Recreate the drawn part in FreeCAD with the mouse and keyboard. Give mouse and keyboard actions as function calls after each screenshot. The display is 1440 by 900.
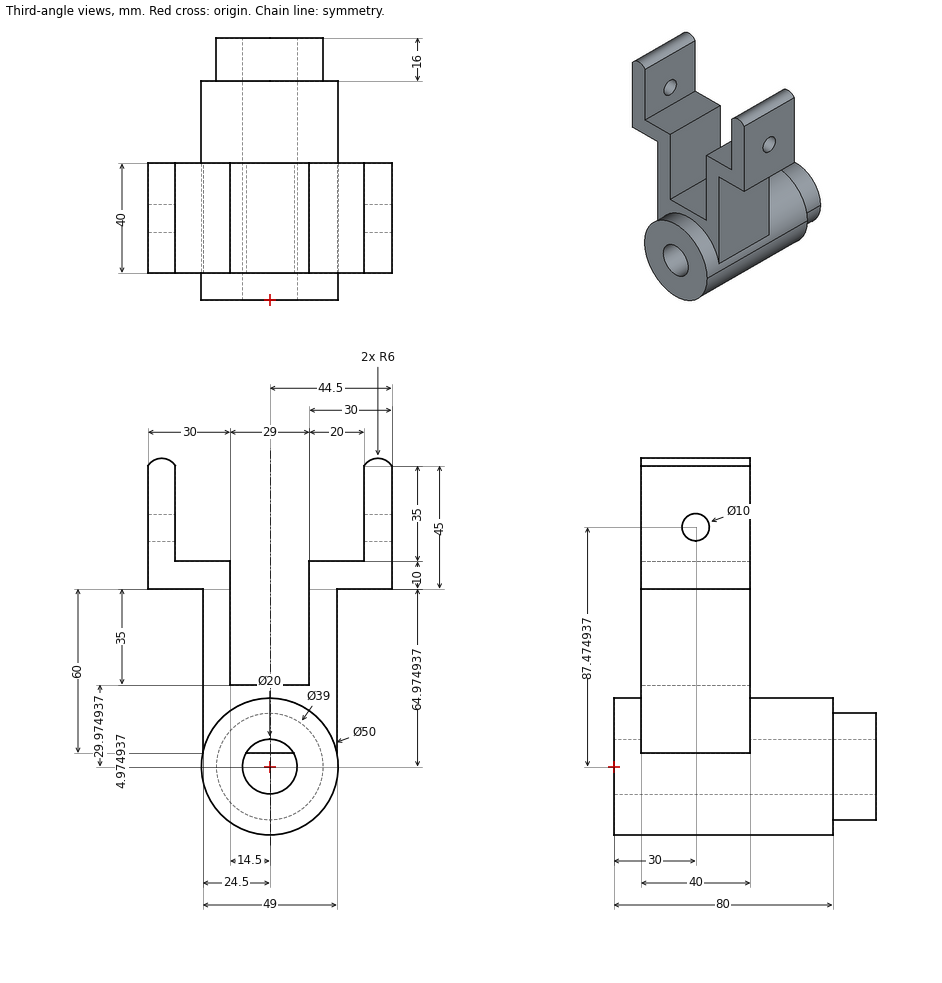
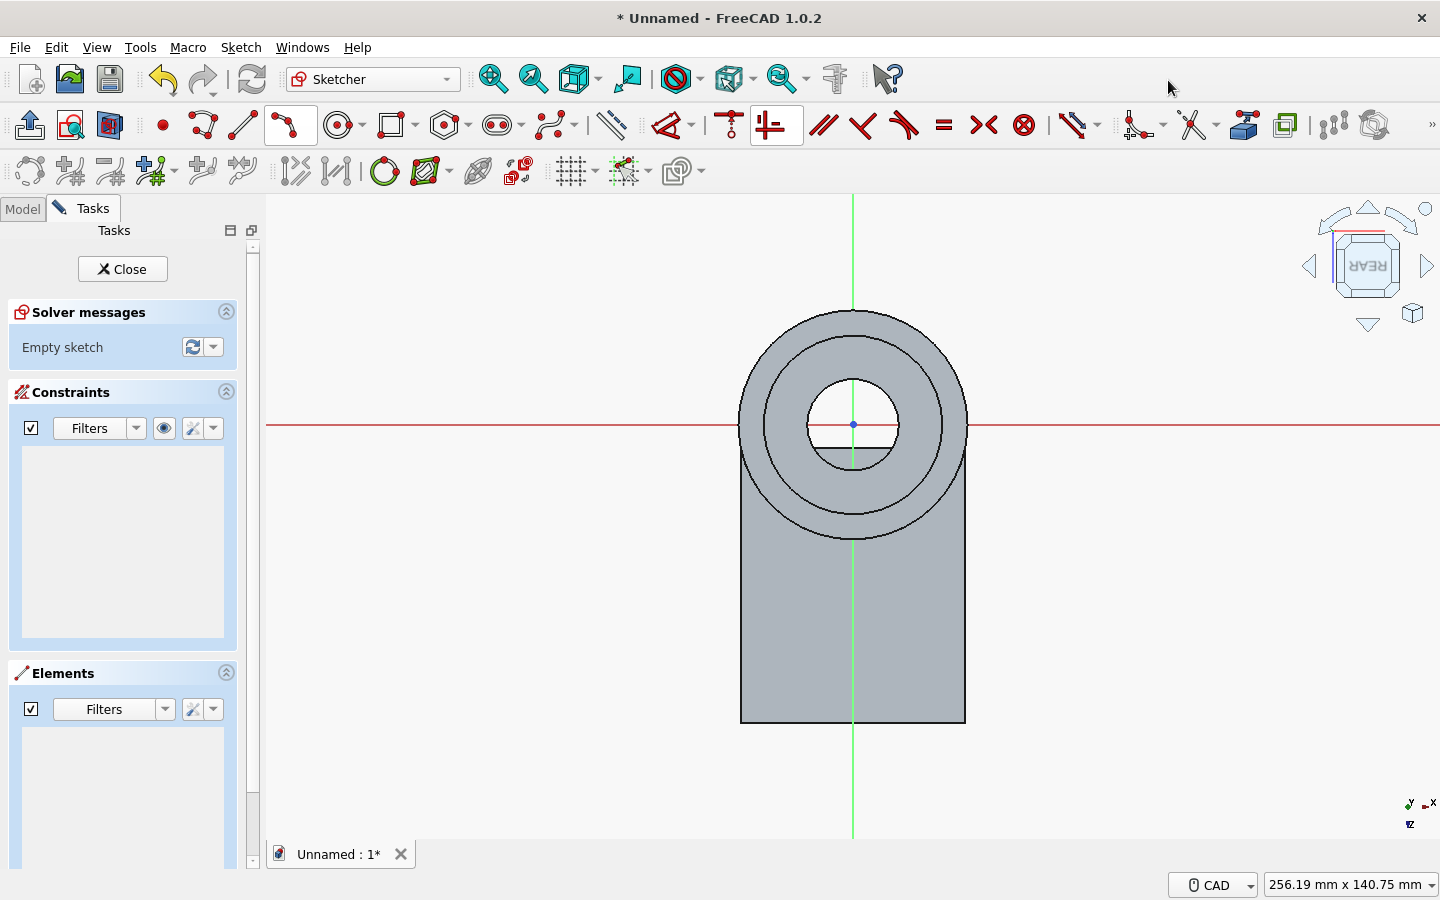
click(110, 126)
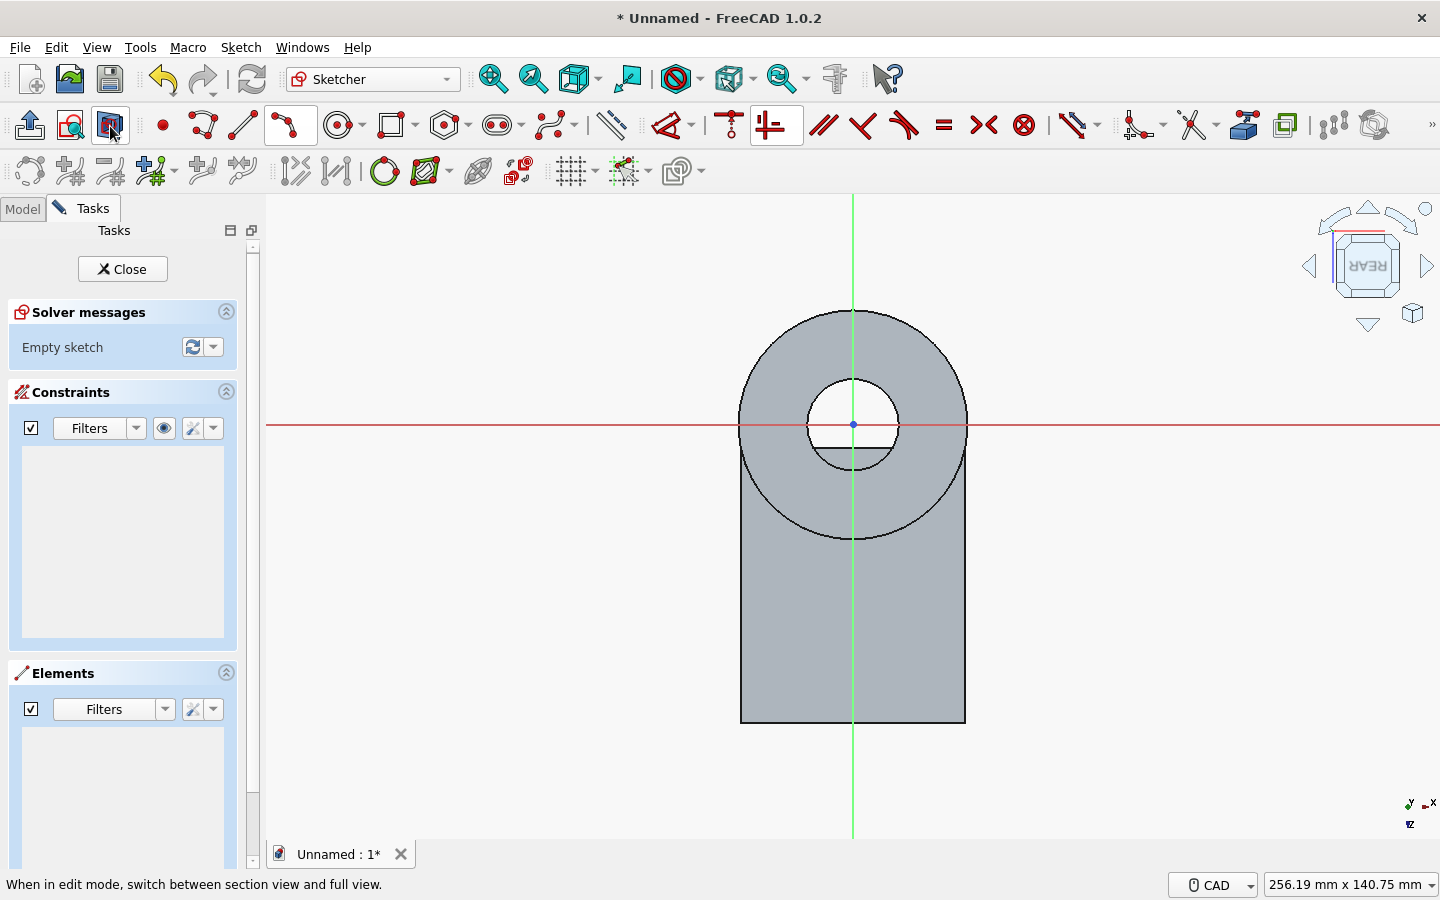
scroll(992, 690, up, 2)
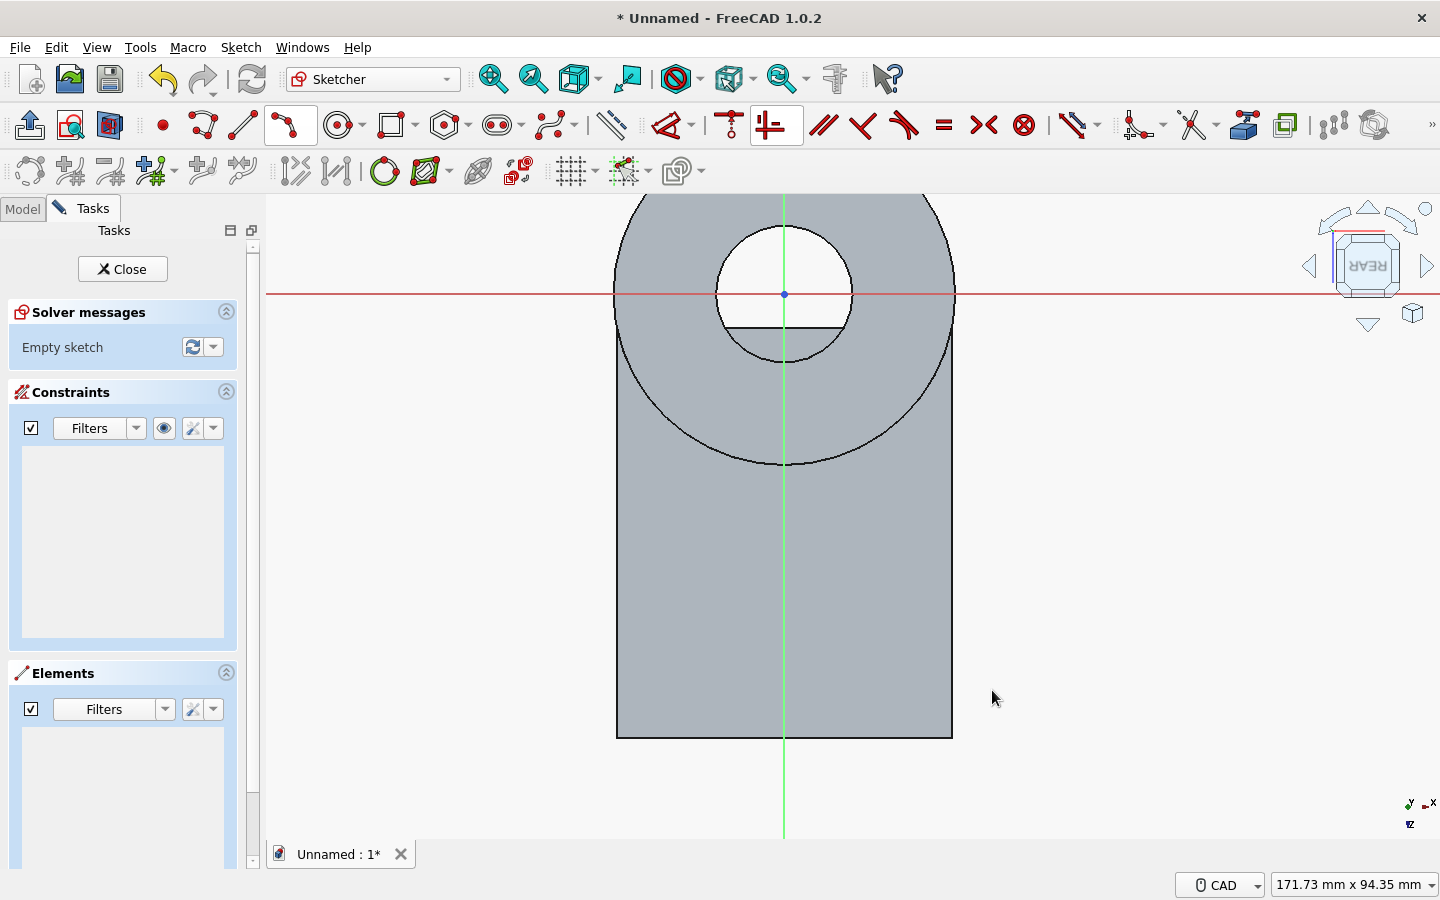
click(392, 126)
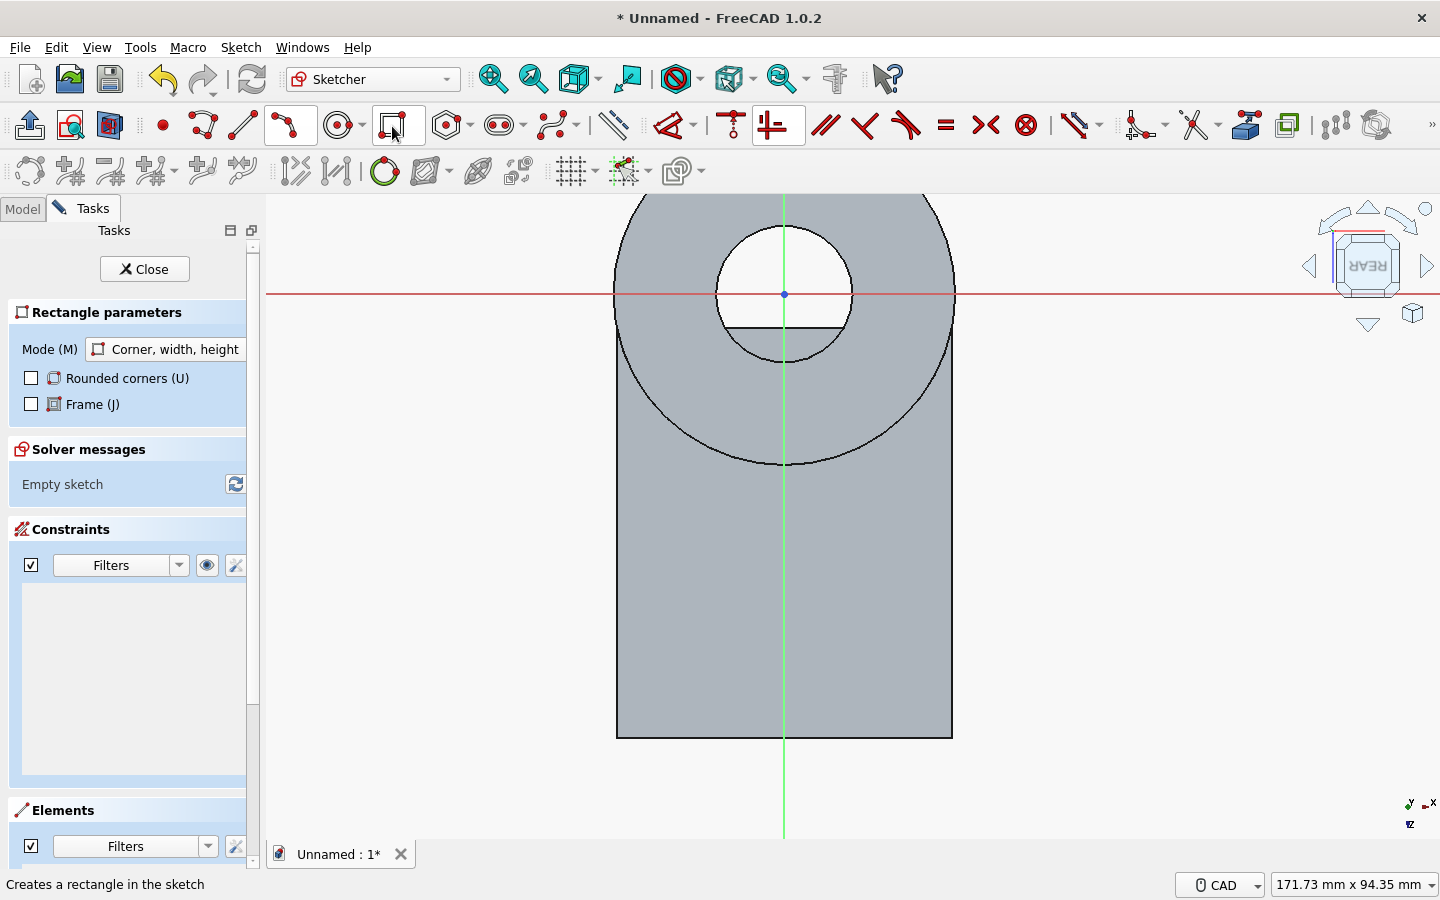
click(685, 499)
click(883, 738)
key(Escape)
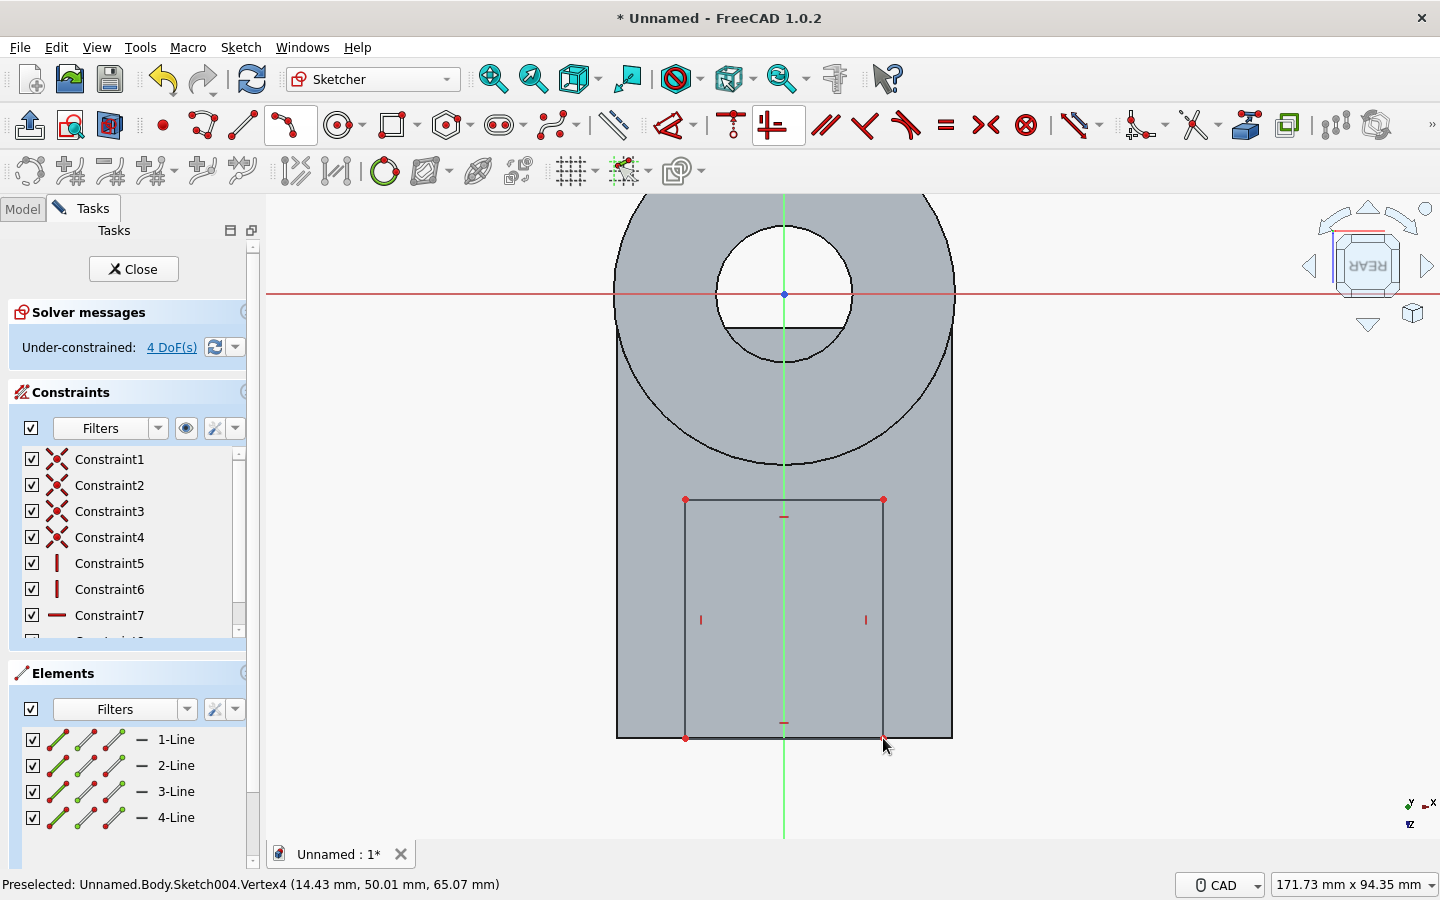
click(668, 126)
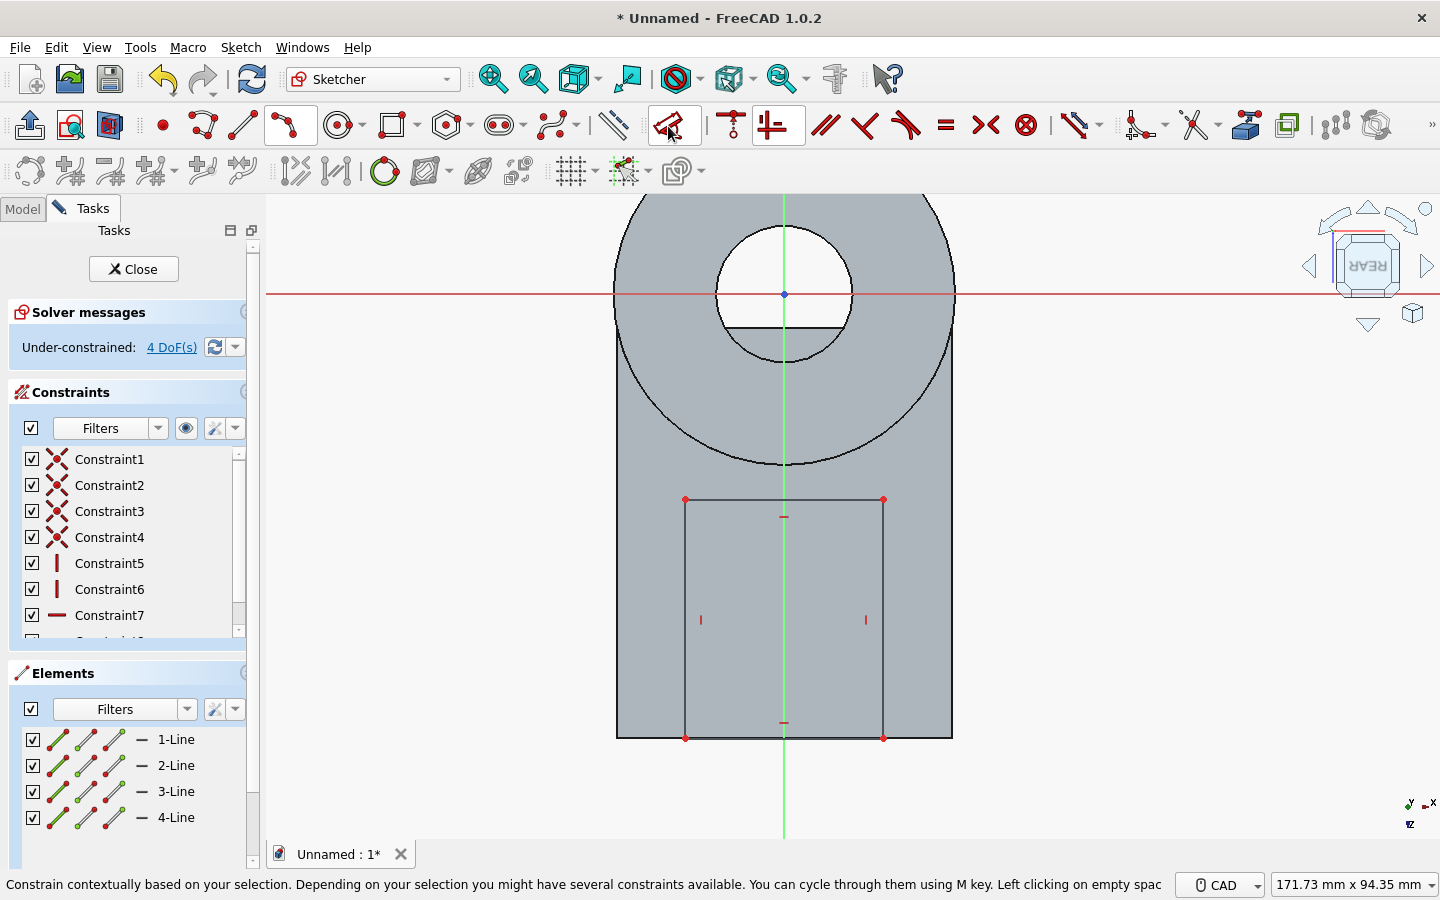
click(685, 572)
click(651, 619)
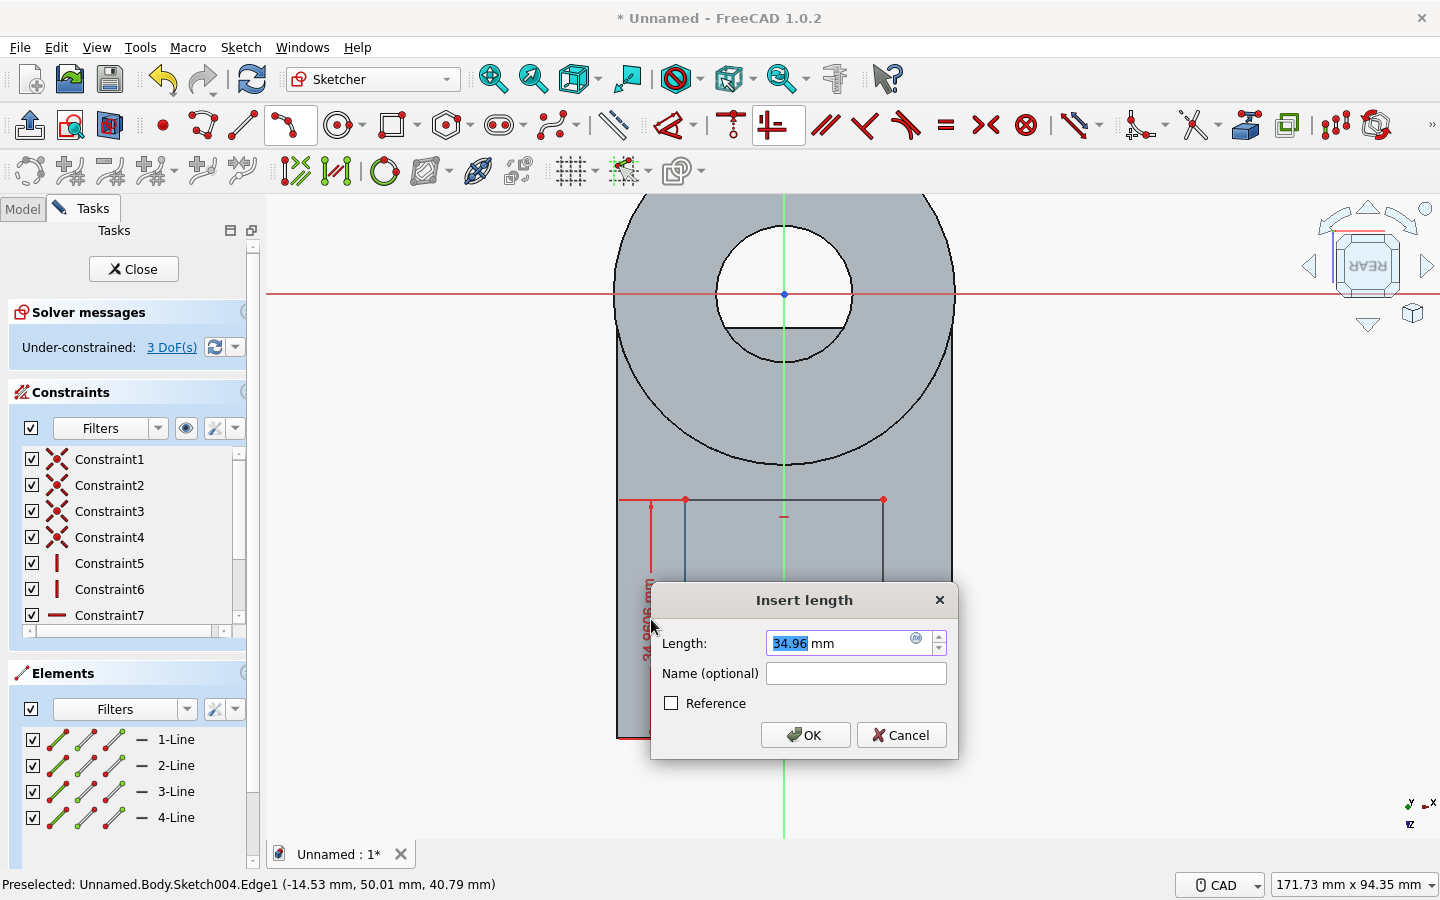
text(35)
key(Return)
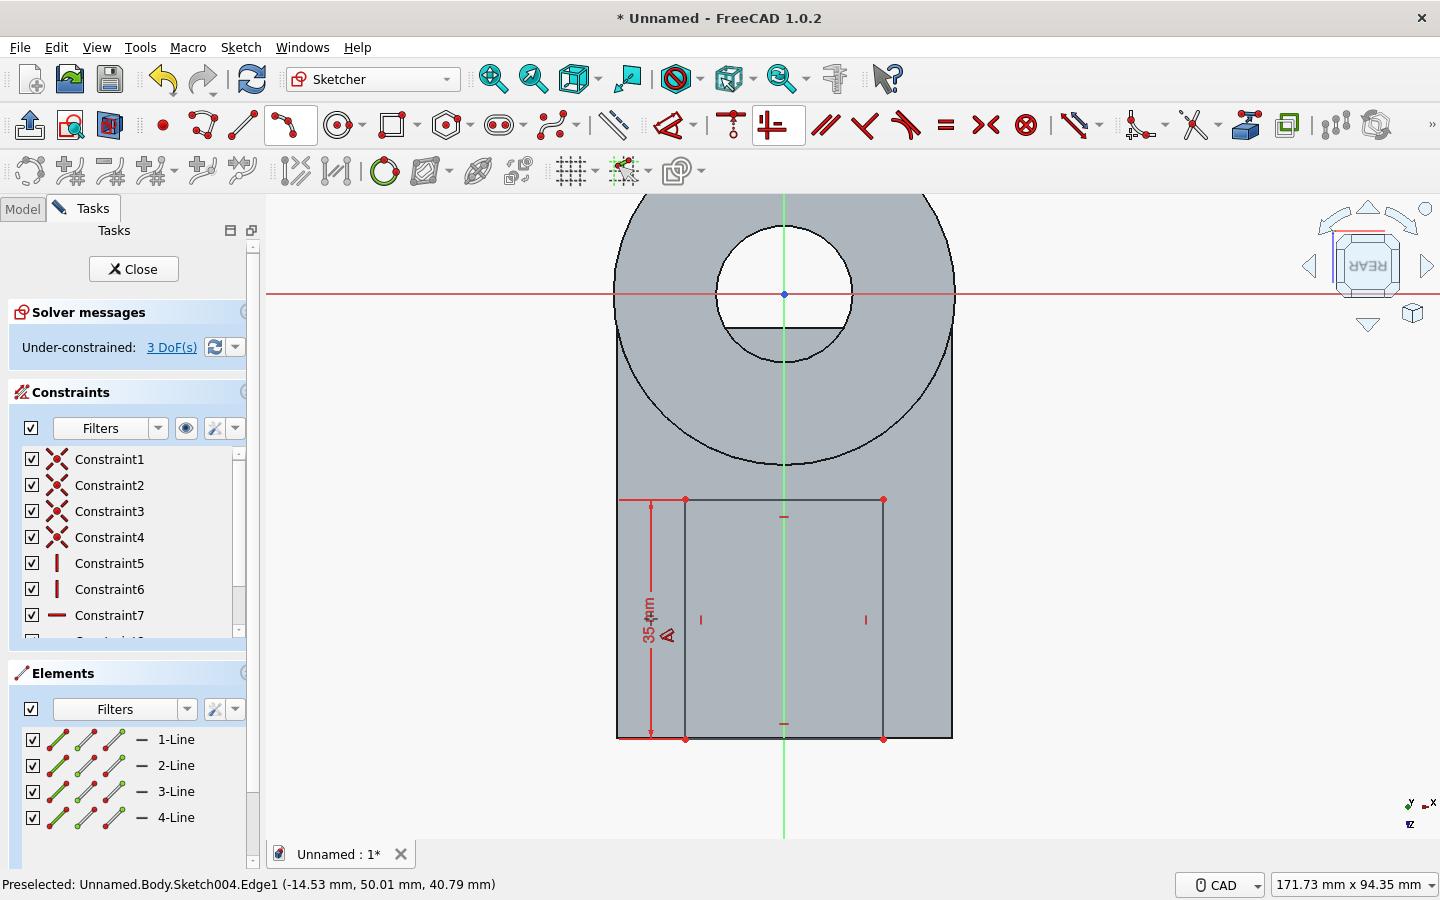
click(744, 739)
click(738, 773)